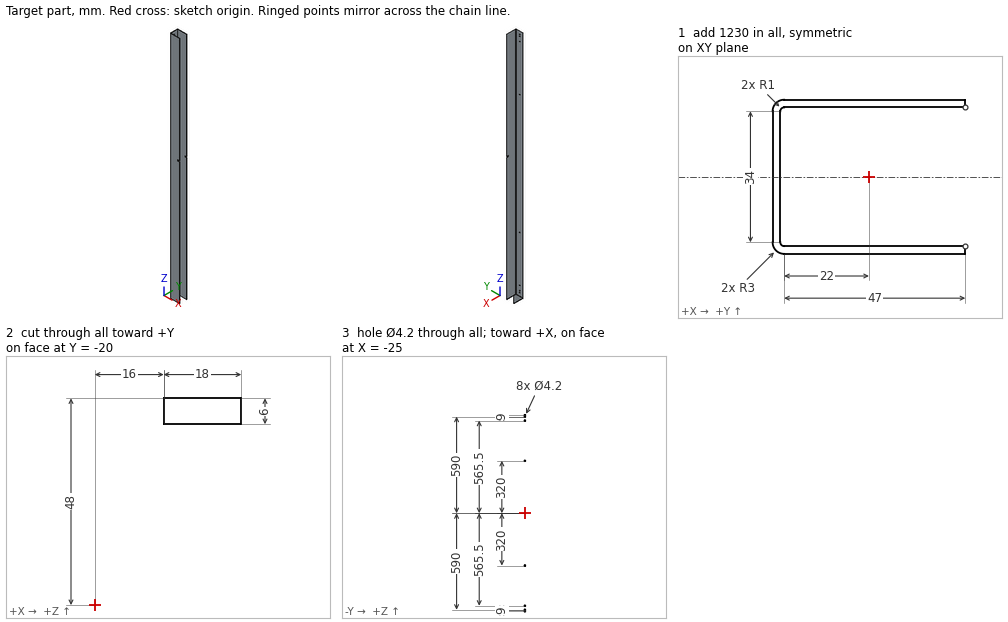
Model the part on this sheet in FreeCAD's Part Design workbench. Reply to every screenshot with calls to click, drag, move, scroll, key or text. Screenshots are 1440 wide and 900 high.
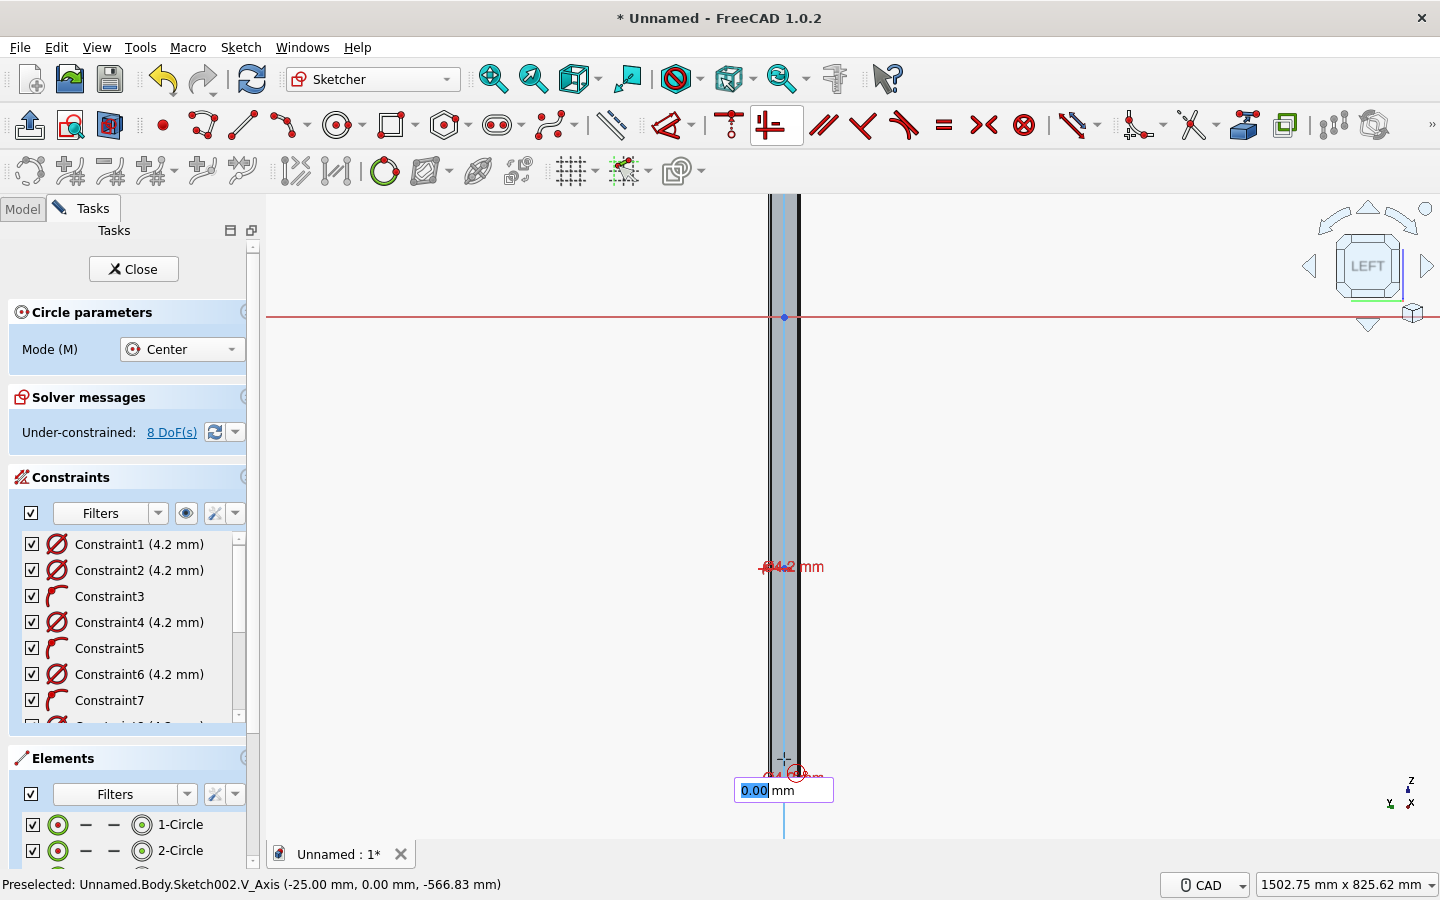
scroll(786, 758, up, 12)
move(780, 754)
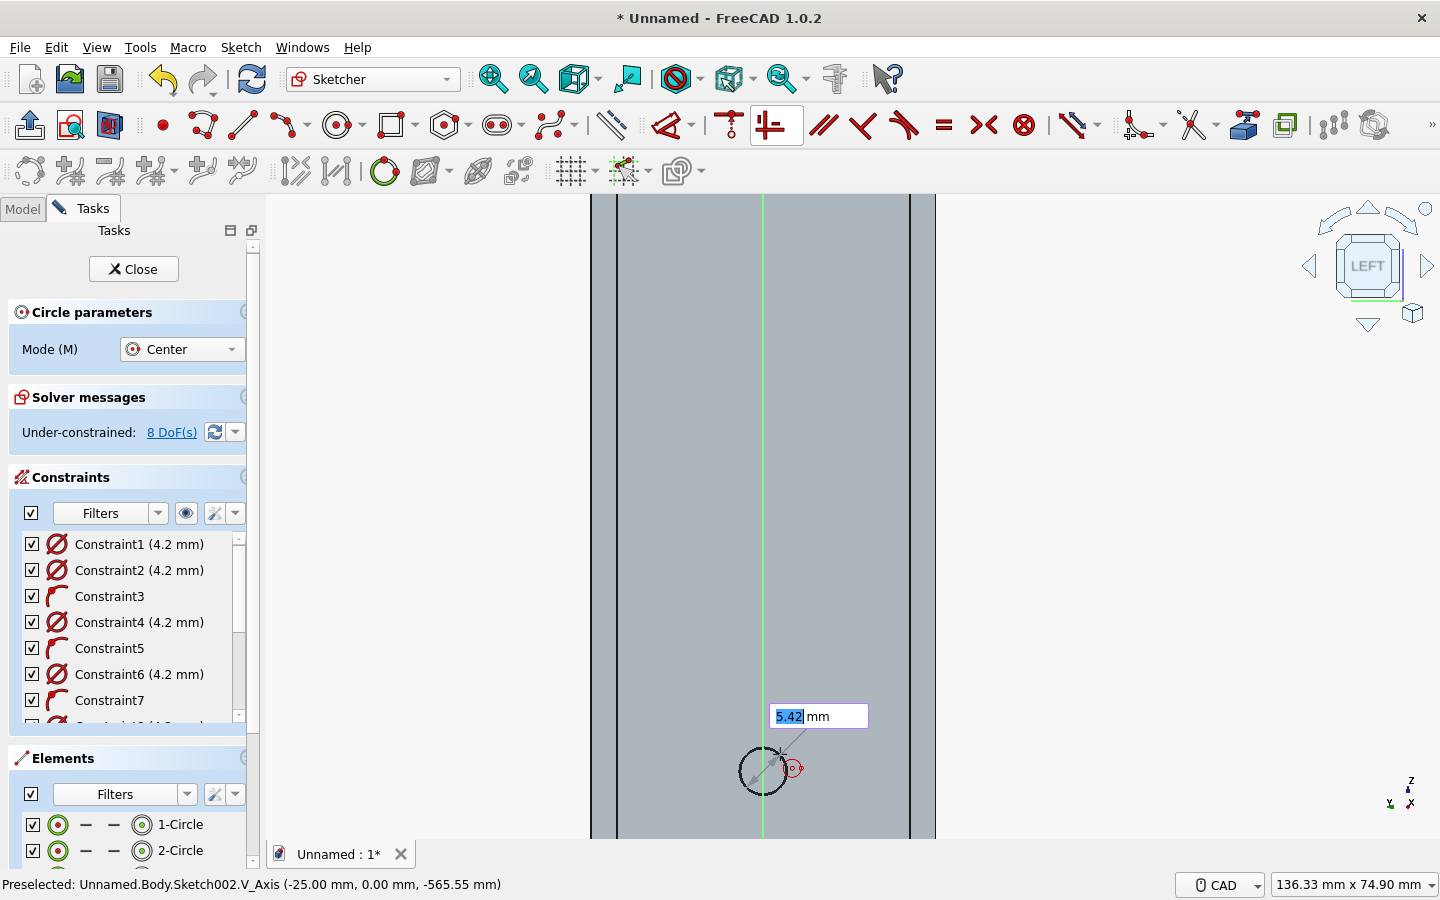
text(4.2)
key(Return)
key(Escape)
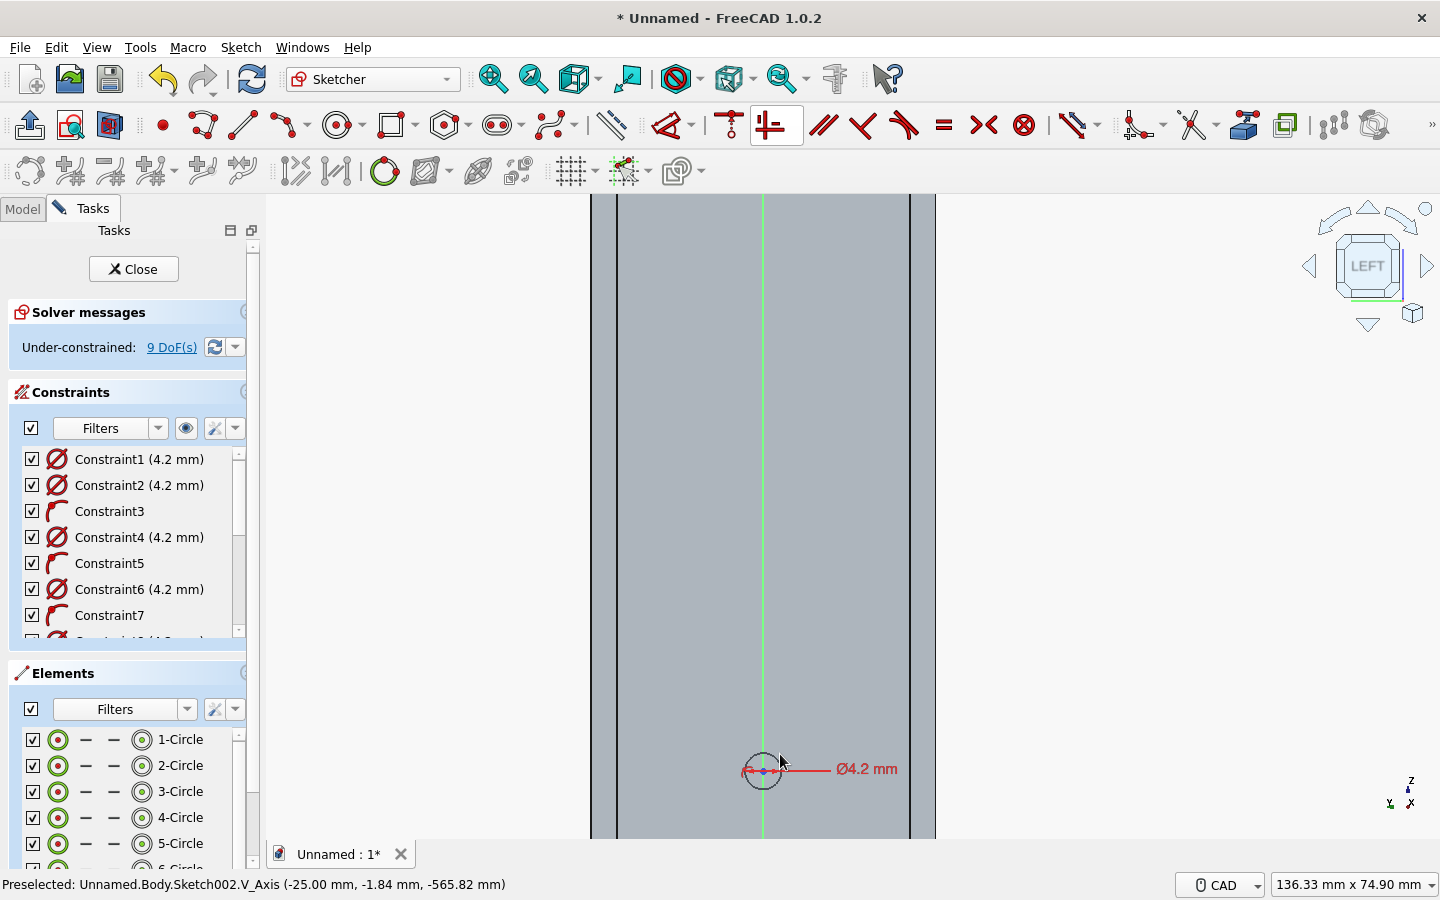
scroll(786, 759, down, 15)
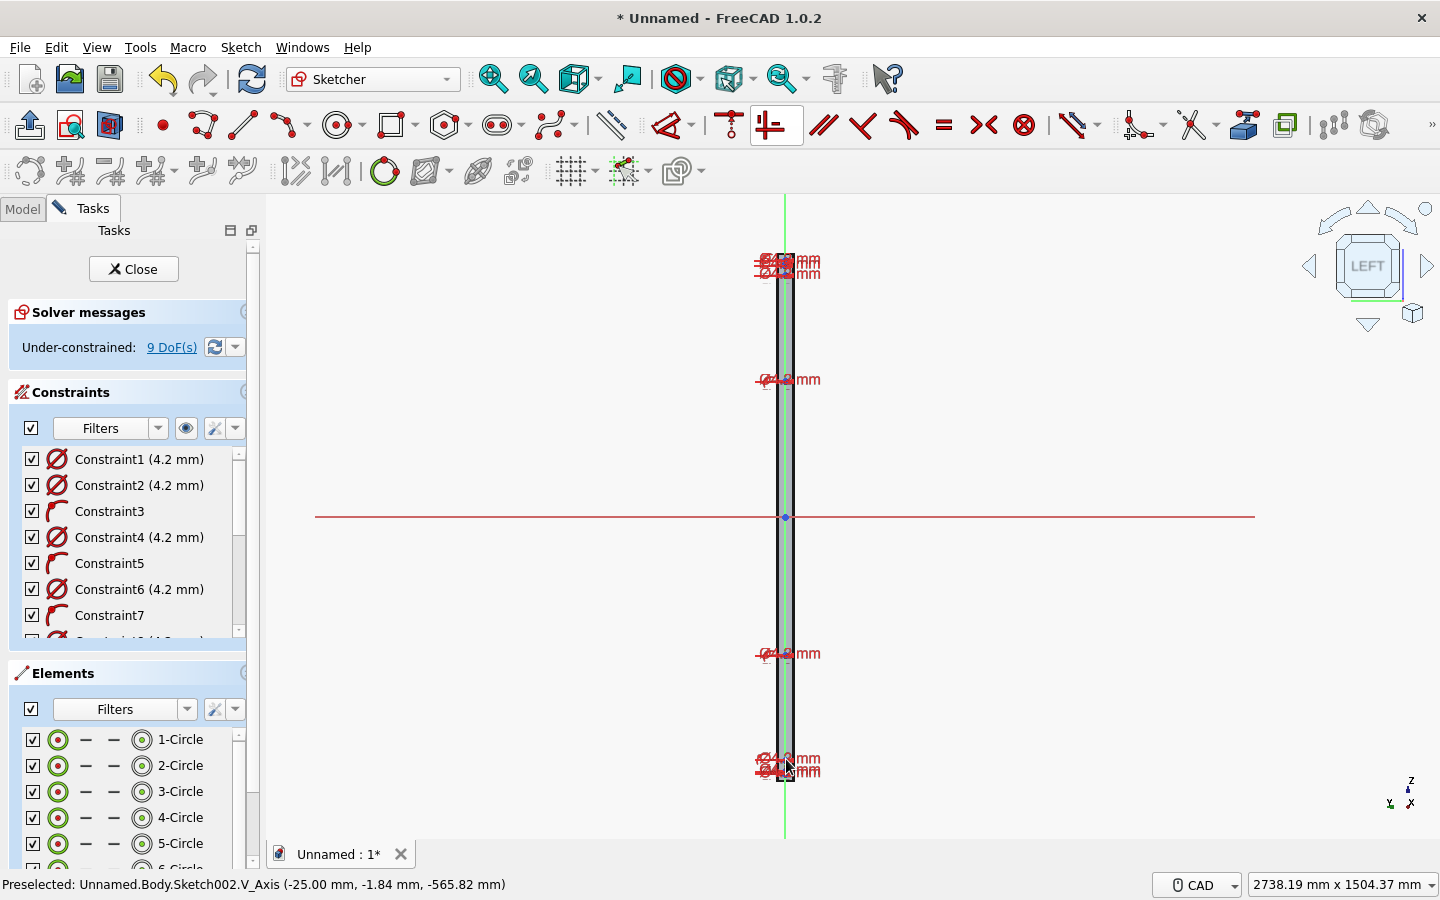
scroll(785, 266, up, 5)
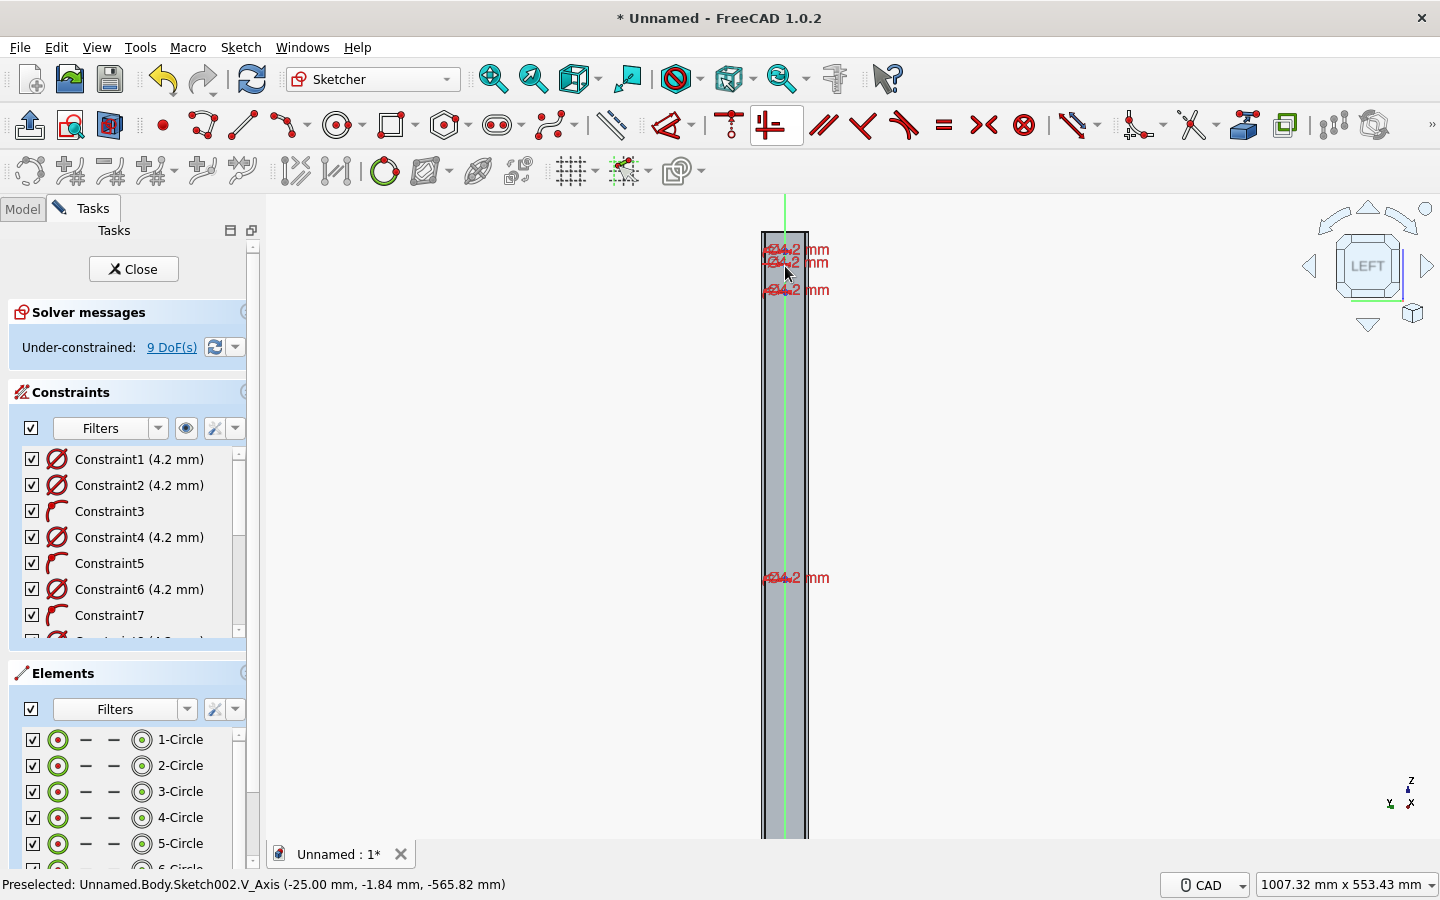
click(784, 264)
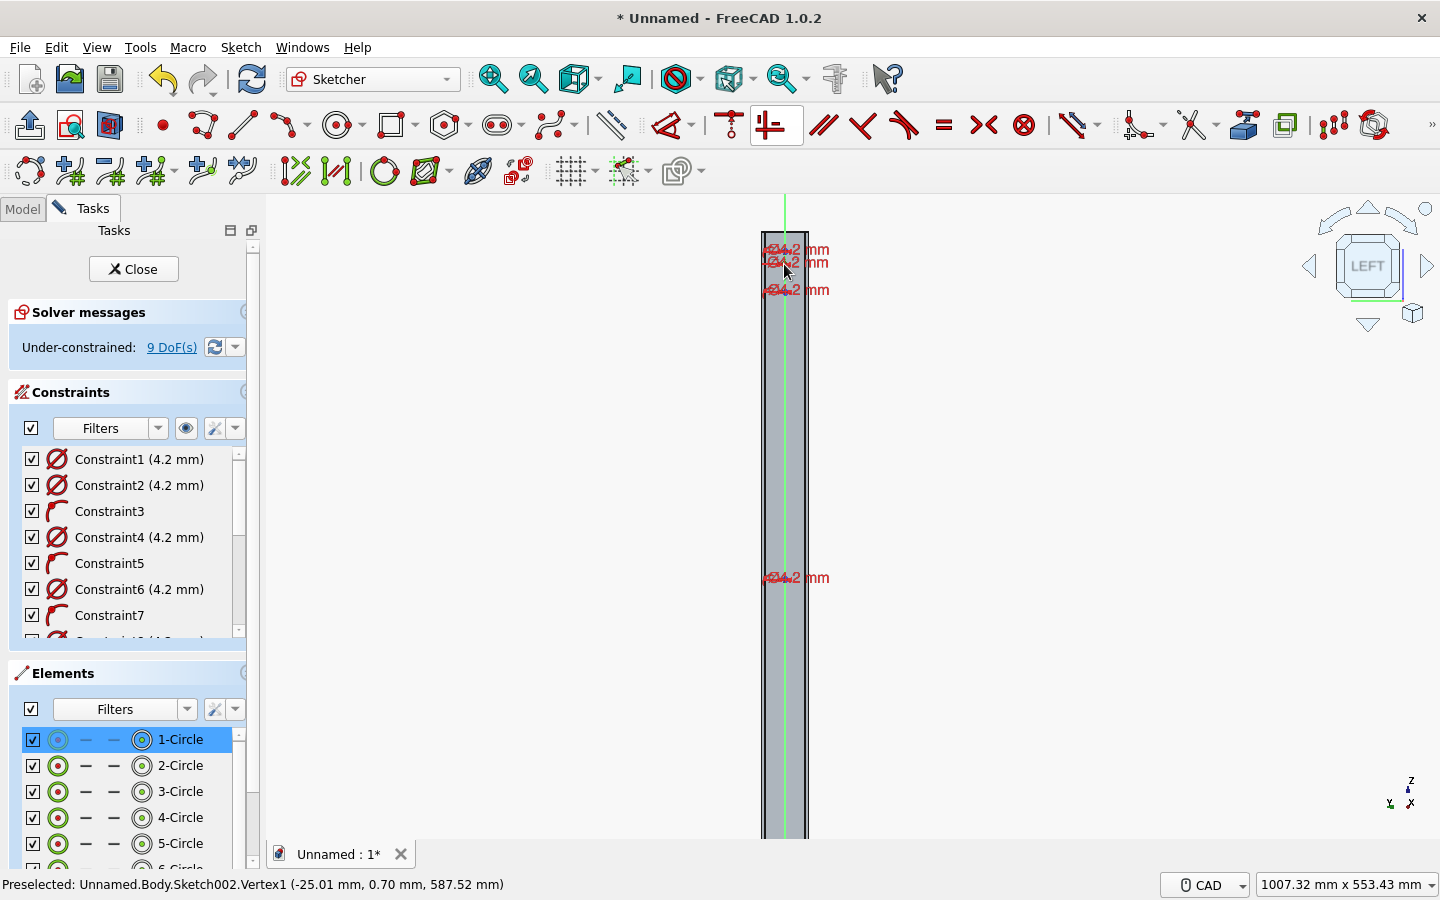
click(785, 769)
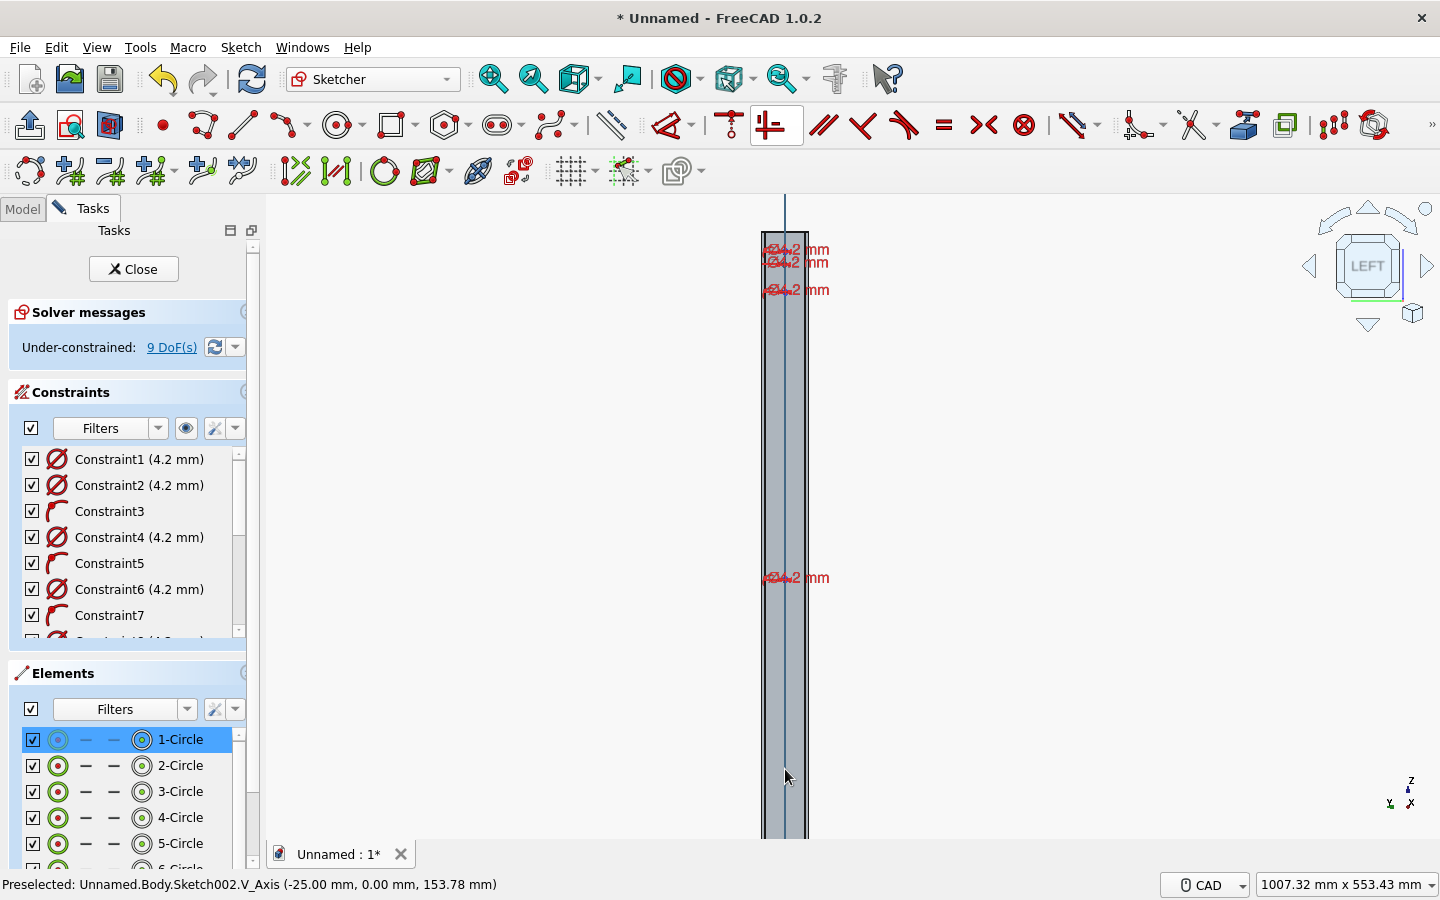
key(c)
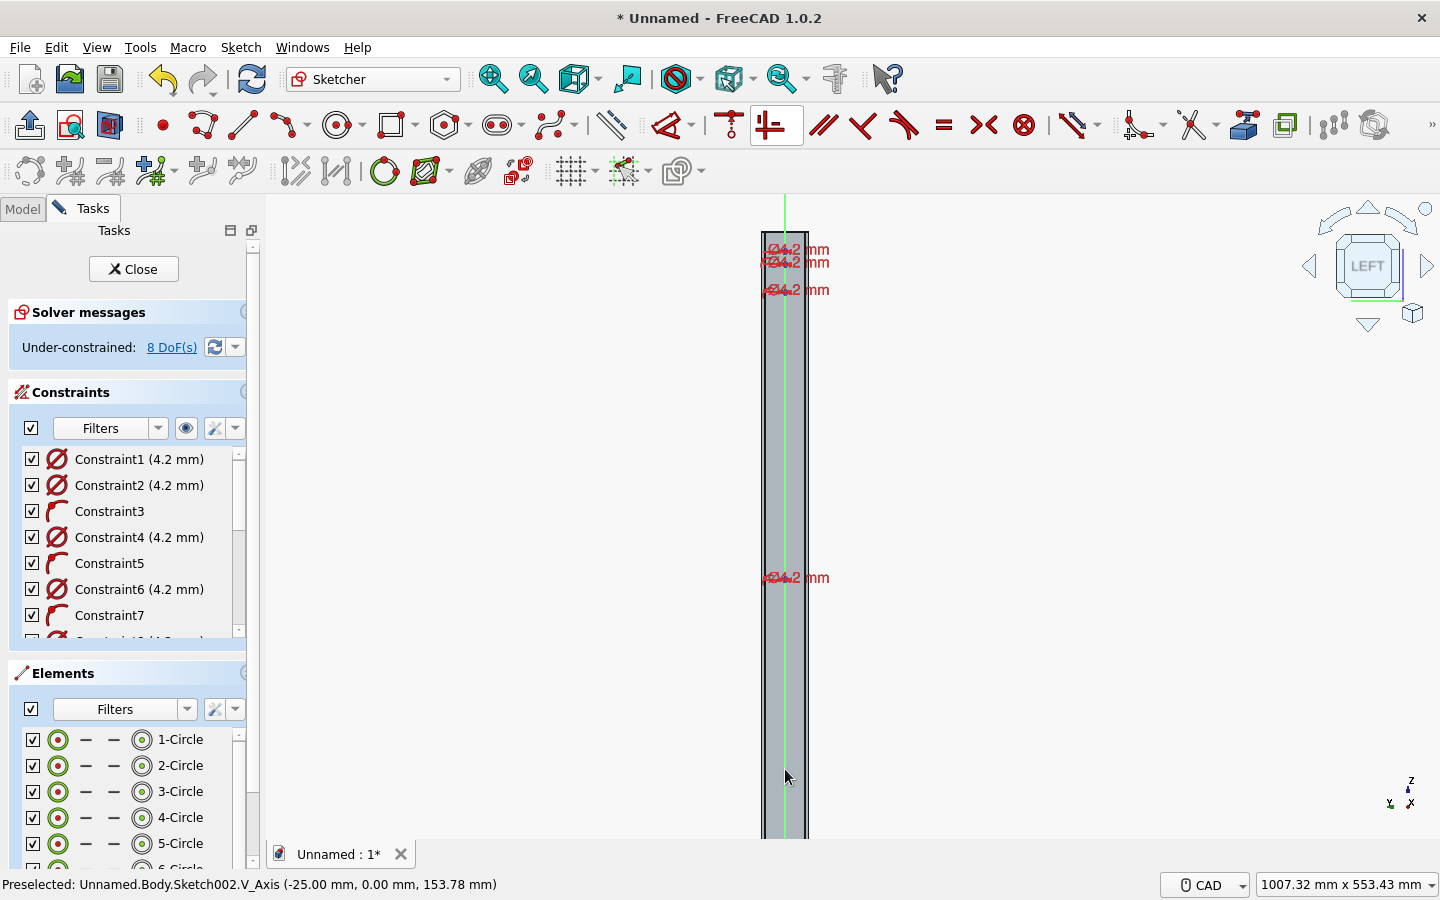
key(d)